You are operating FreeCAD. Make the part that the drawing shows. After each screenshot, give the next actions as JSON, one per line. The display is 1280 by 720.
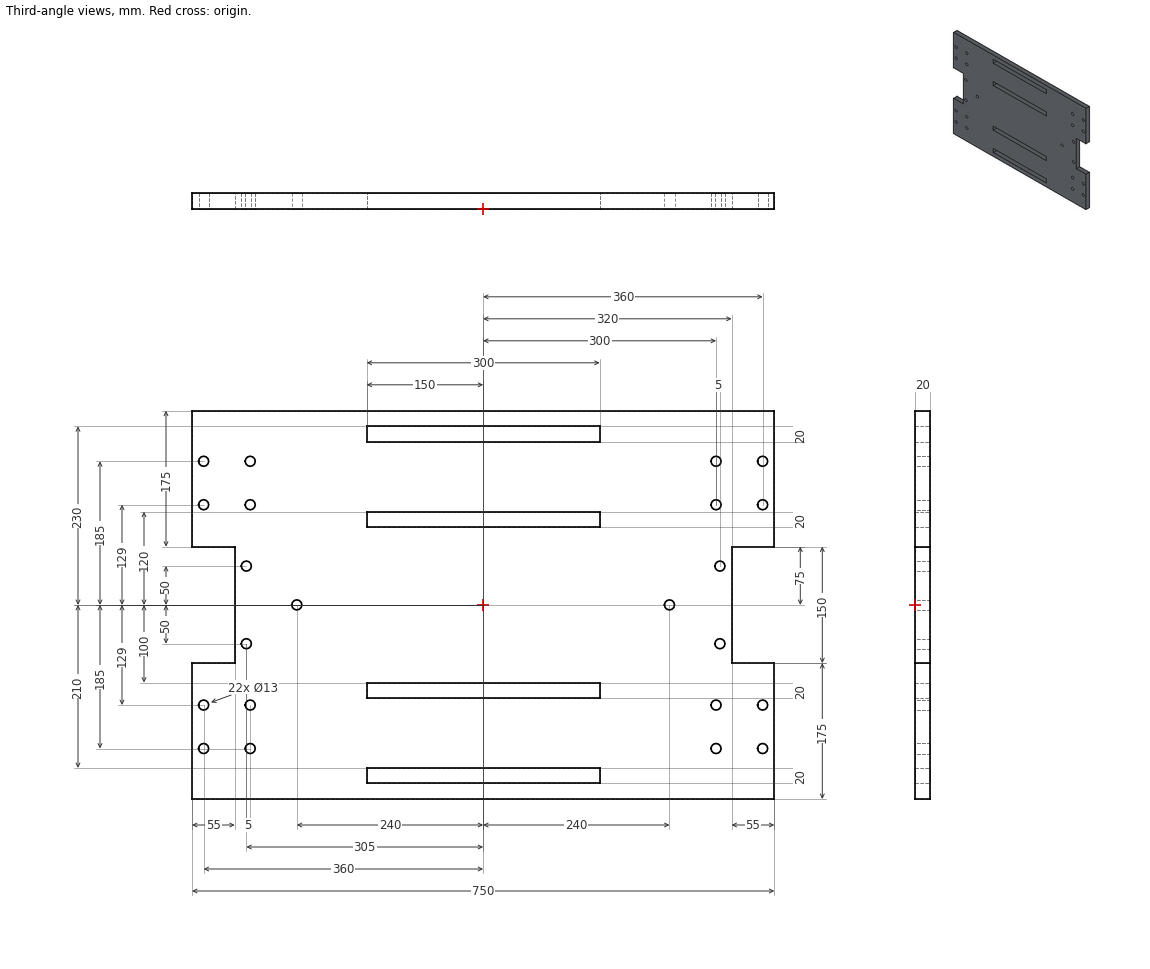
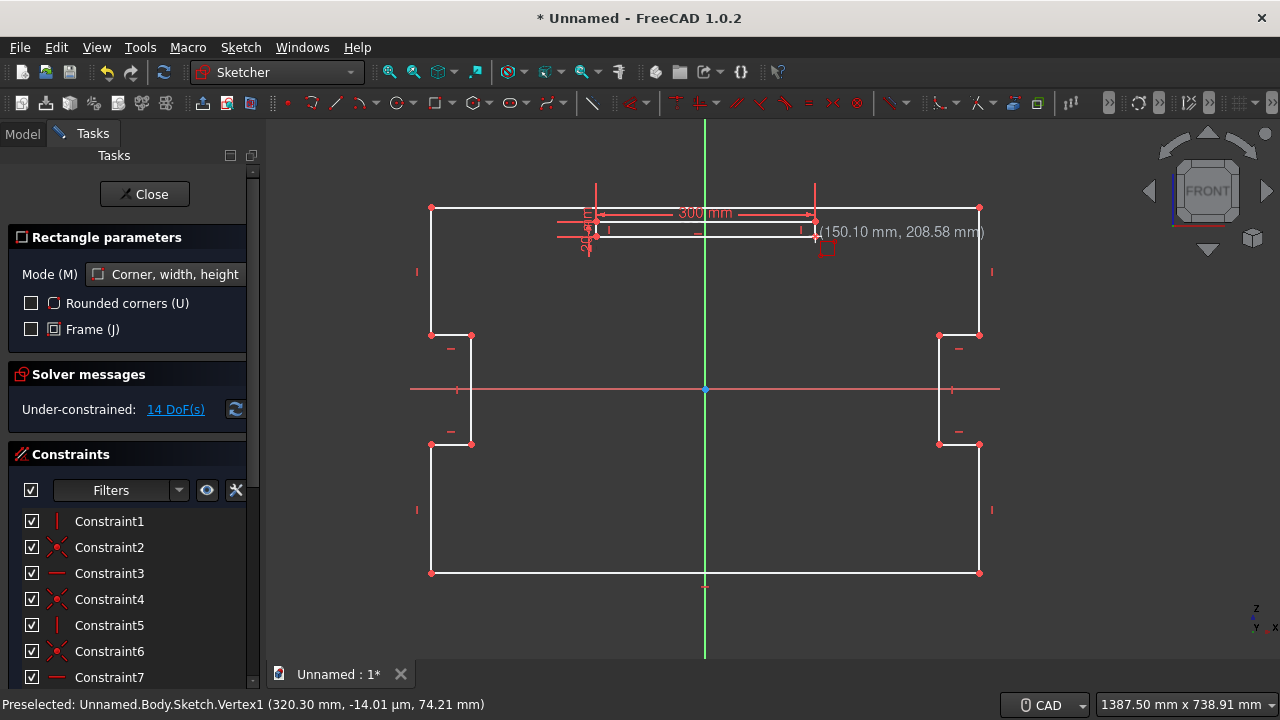
{"action": "left_click", "coordinate": [596, 302]}
{"action": "mouse_move", "coordinate": [815, 316]}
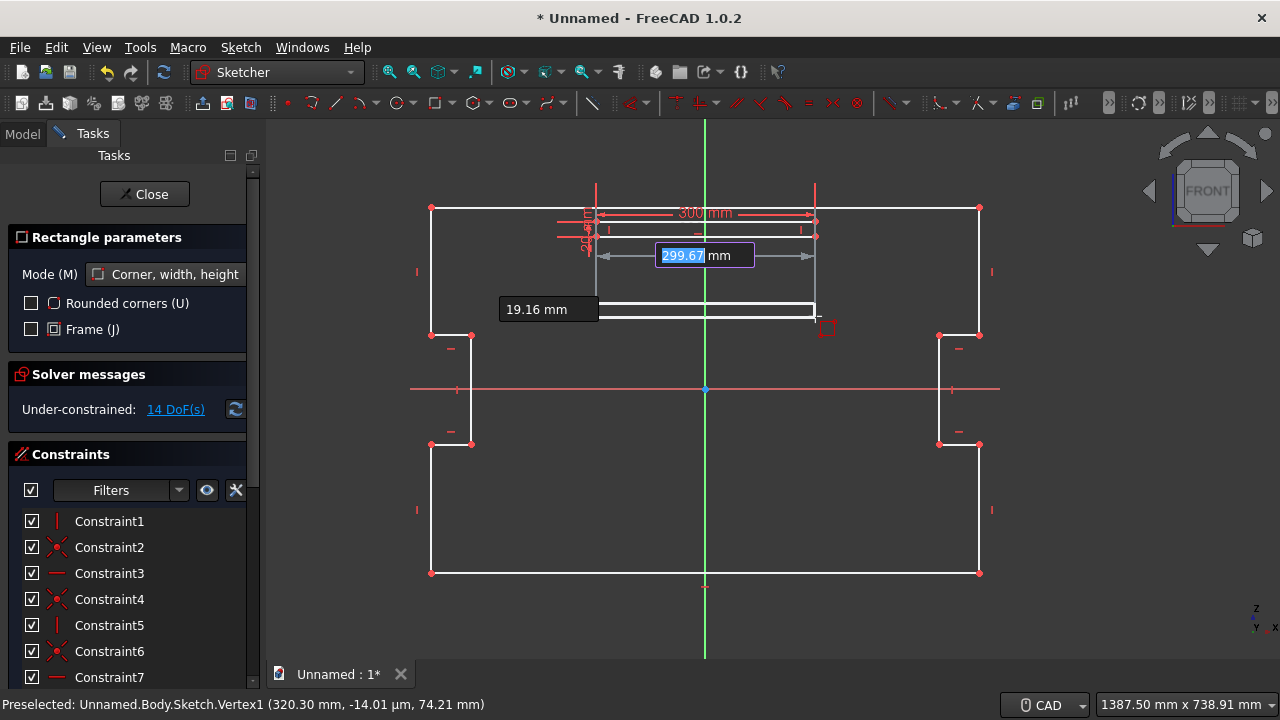
{"action": "type", "text": "300"}
{"action": "key", "text": "Tab"}
{"action": "type", "text": "20"}
{"action": "key", "text": "Return"}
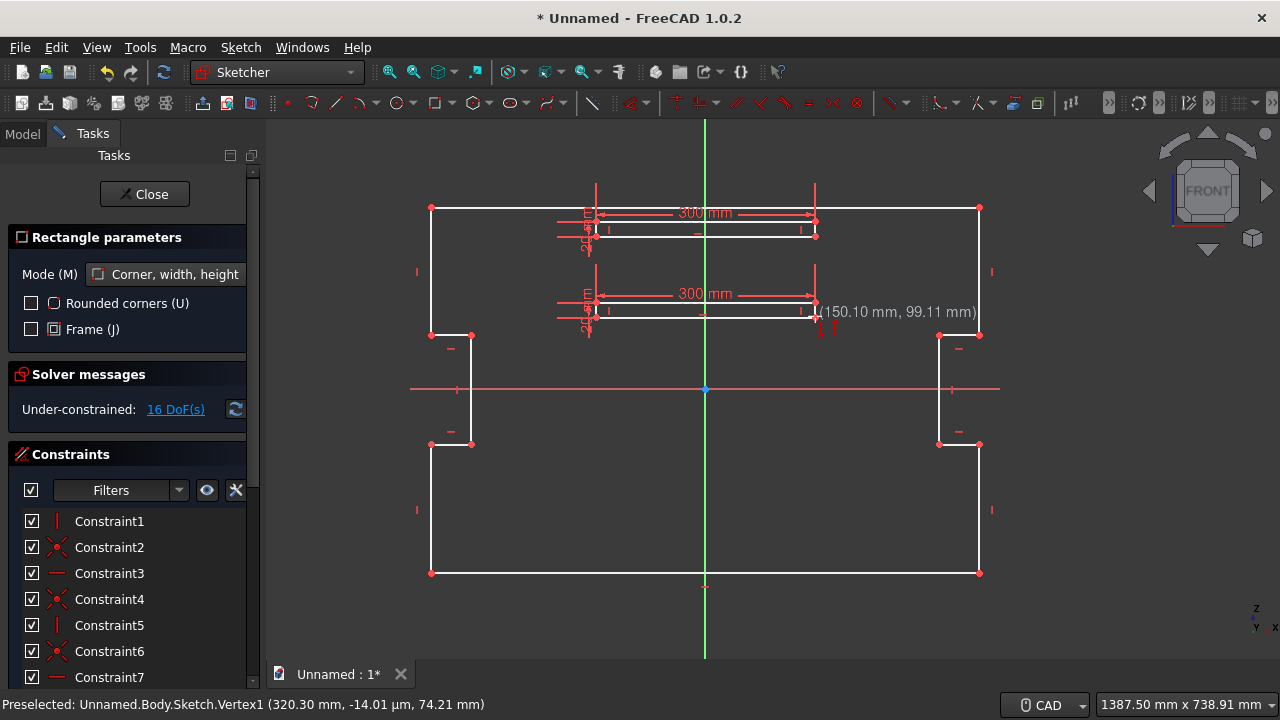
{"action": "left_click", "coordinate": [596, 463]}
{"action": "mouse_move", "coordinate": [815, 477]}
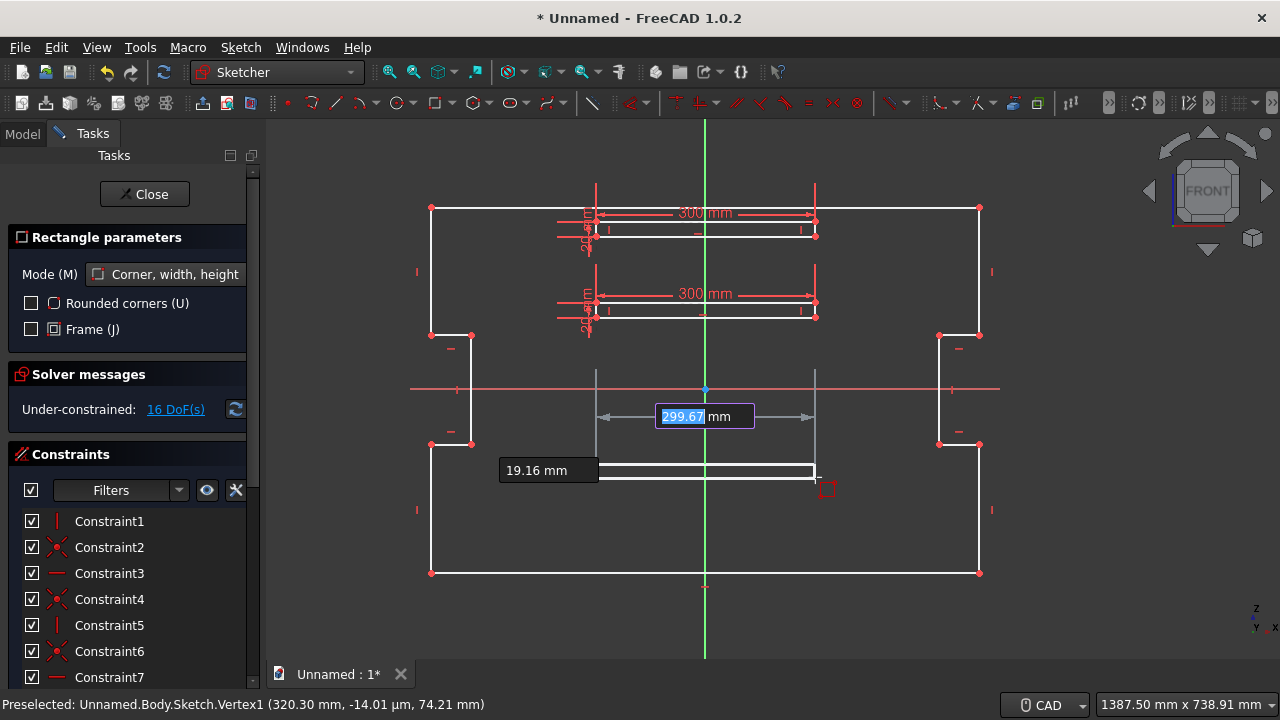
{"action": "type", "text": "300"}
{"action": "key", "text": "Tab"}
{"action": "type", "text": "20"}
{"action": "key", "text": "Return"}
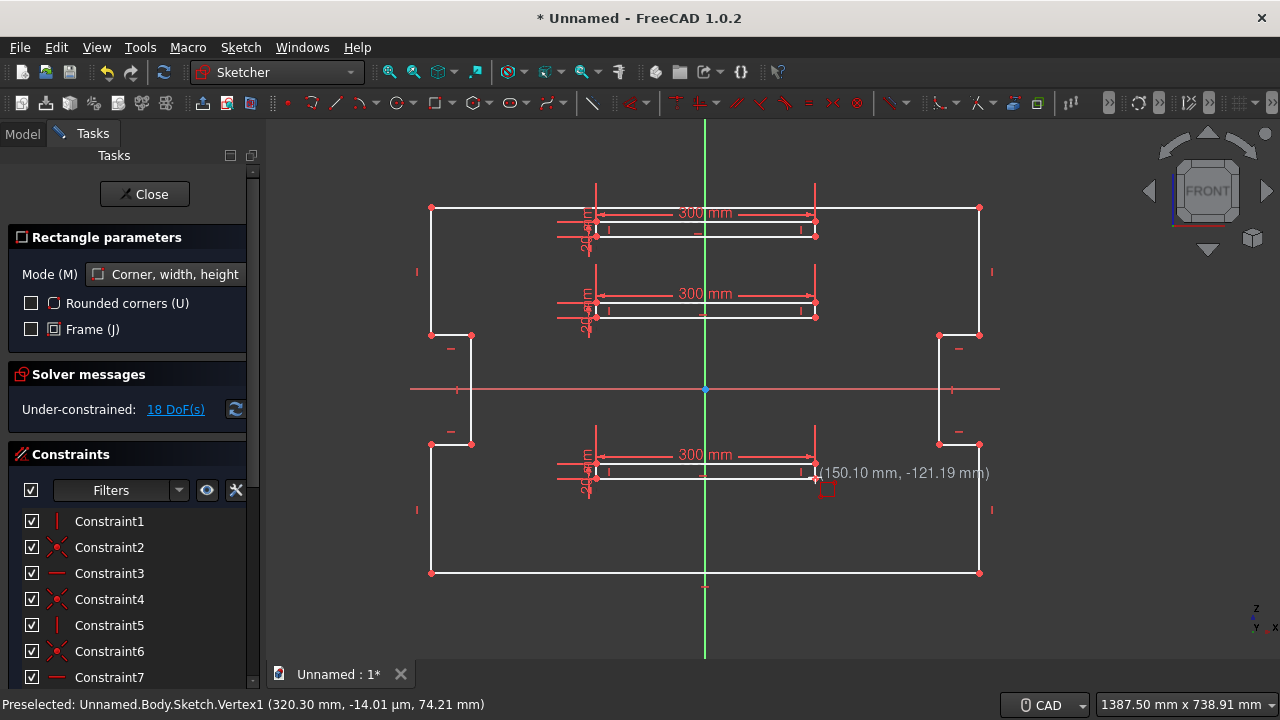
{"action": "left_click", "coordinate": [596, 543]}
{"action": "mouse_move", "coordinate": [815, 558]}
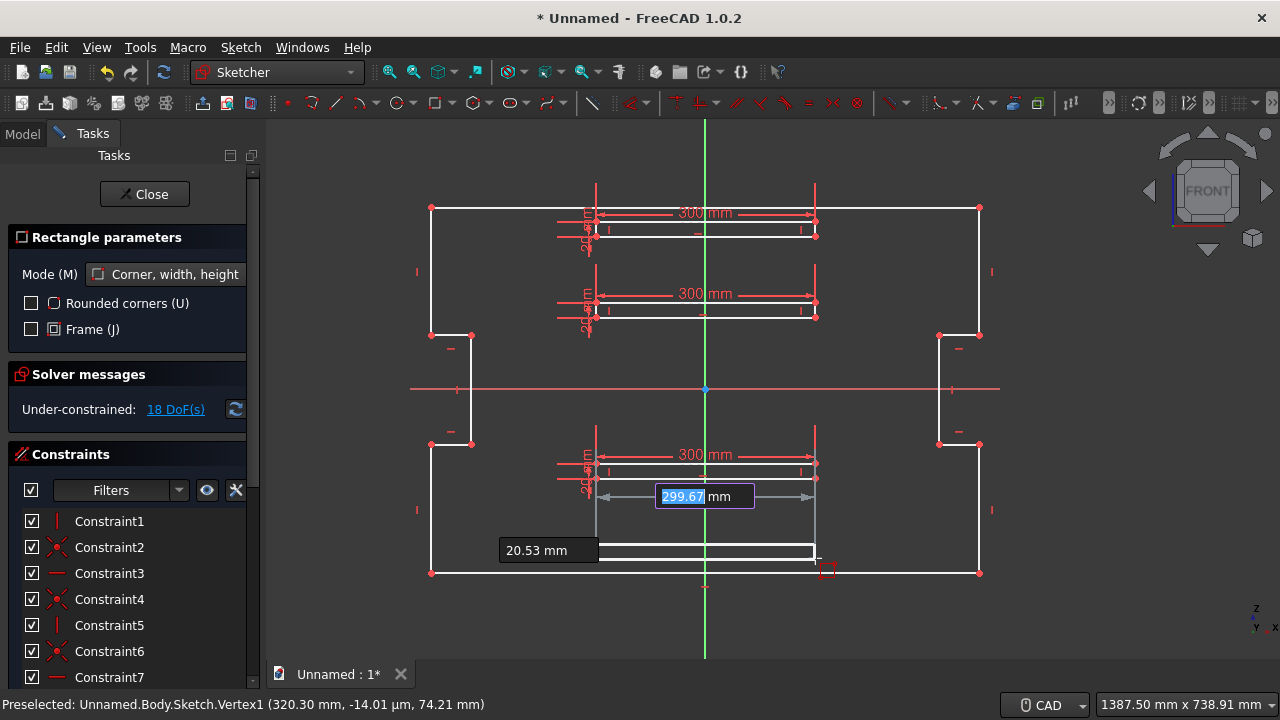
{"action": "type", "text": "300"}
{"action": "key", "text": "Tab"}
{"action": "type", "text": "20"}
{"action": "key", "text": "Return"}
{"action": "key", "text": "Escape"}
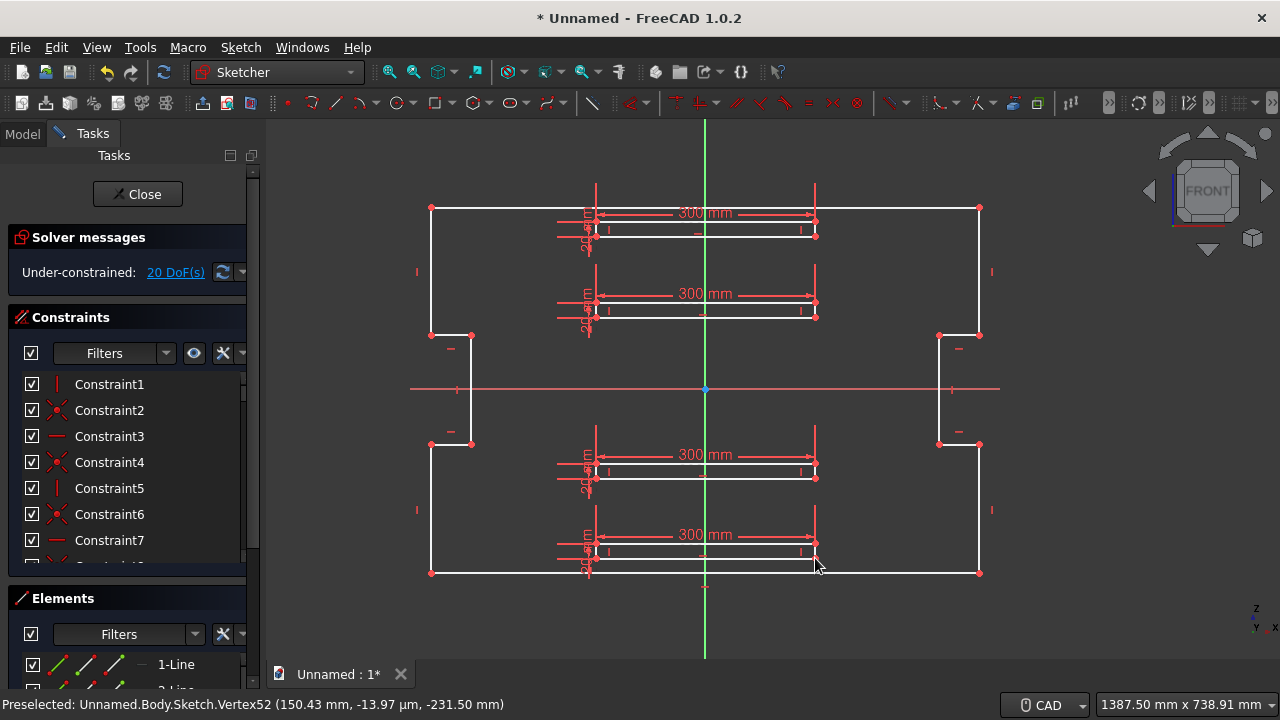
{"action": "left_click", "coordinate": [951, 445]}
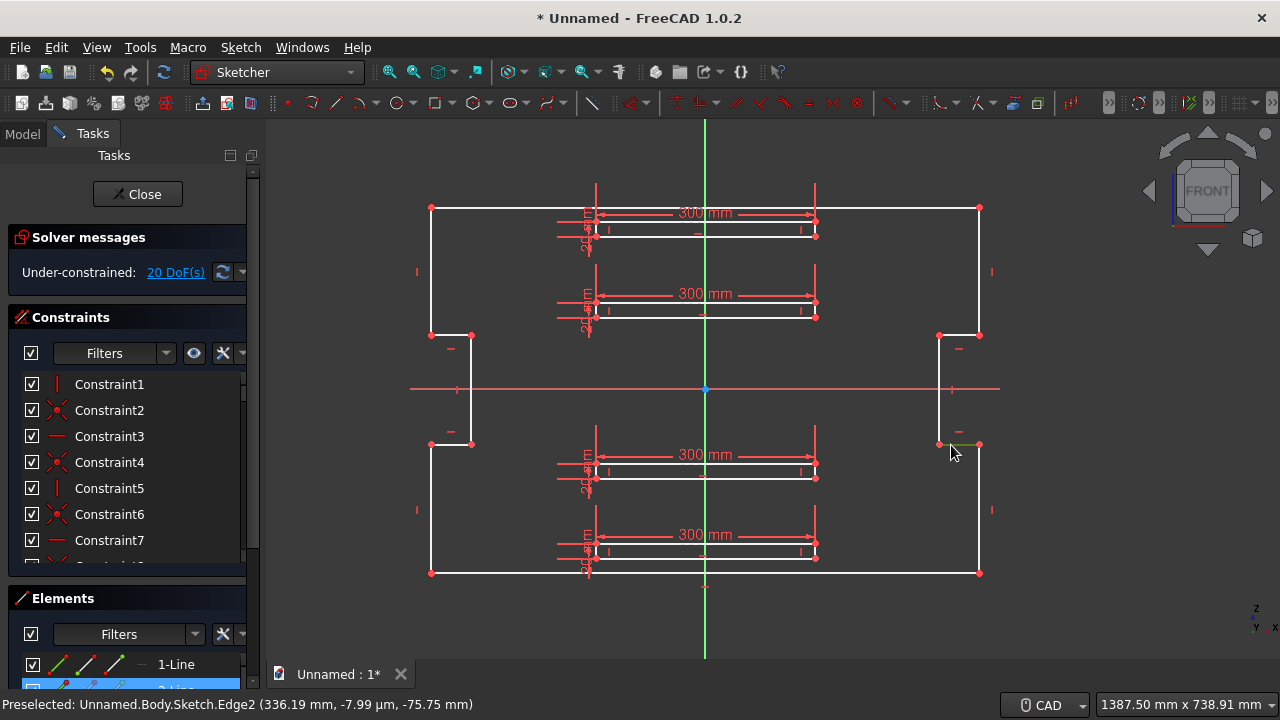
{"action": "key", "text": "l"}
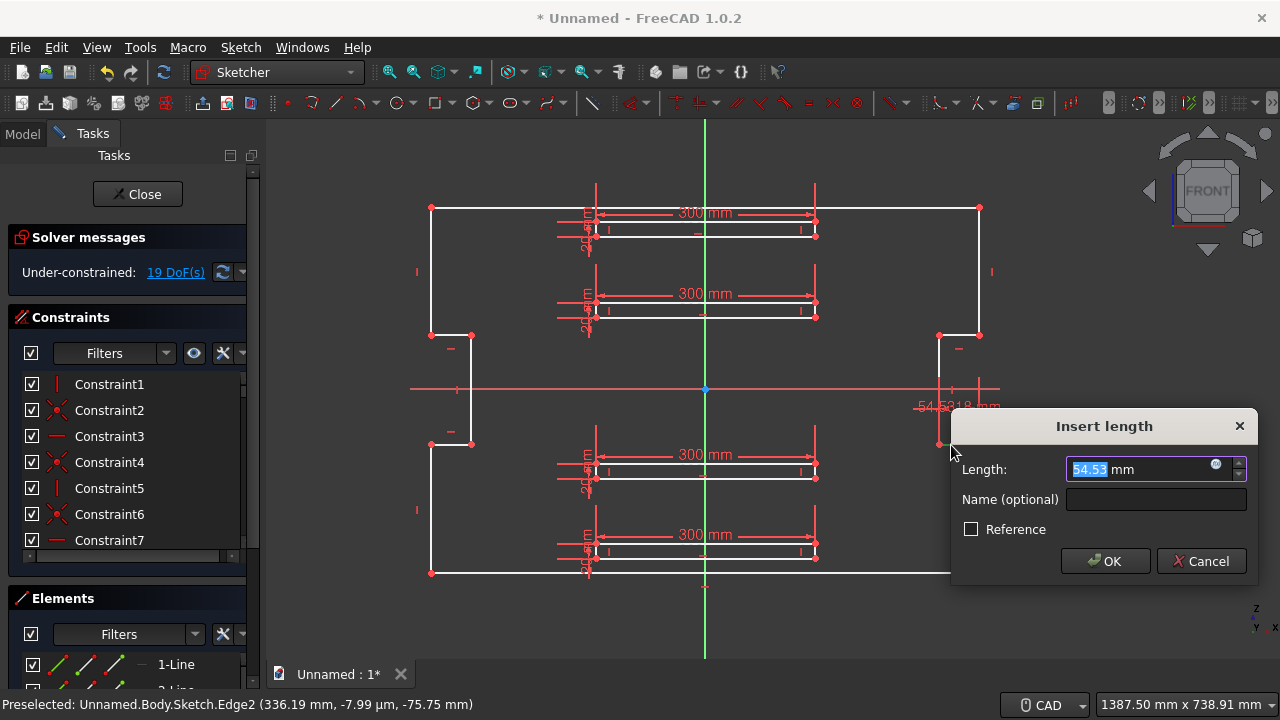
{"action": "type", "text": "55"}
{"action": "key", "text": "Return"}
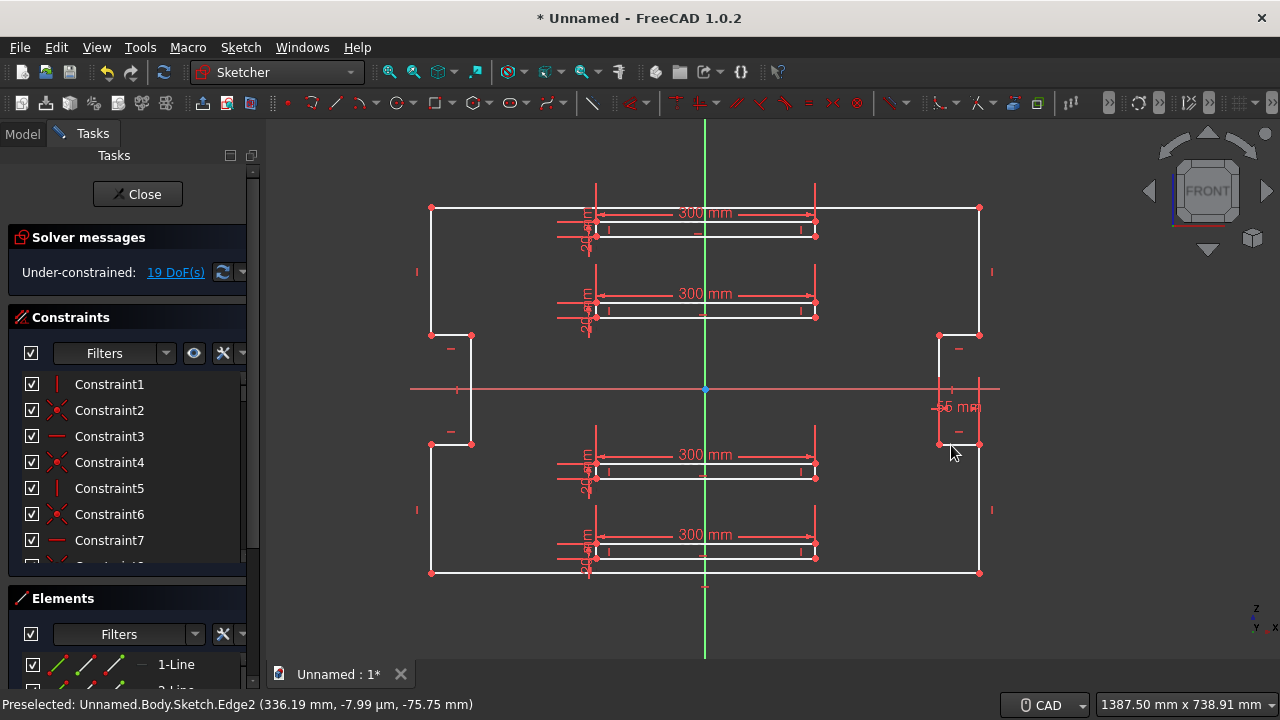
{"action": "left_click", "coordinate": [443, 445]}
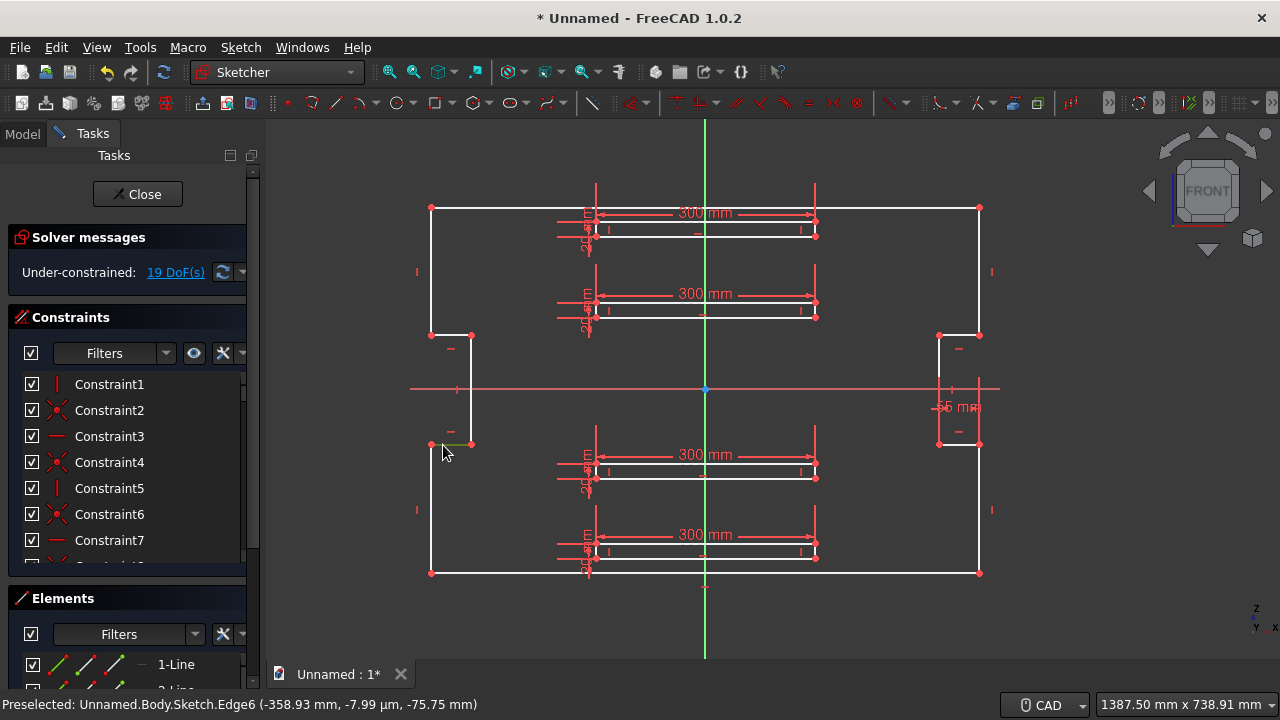
{"action": "key", "text": "l"}